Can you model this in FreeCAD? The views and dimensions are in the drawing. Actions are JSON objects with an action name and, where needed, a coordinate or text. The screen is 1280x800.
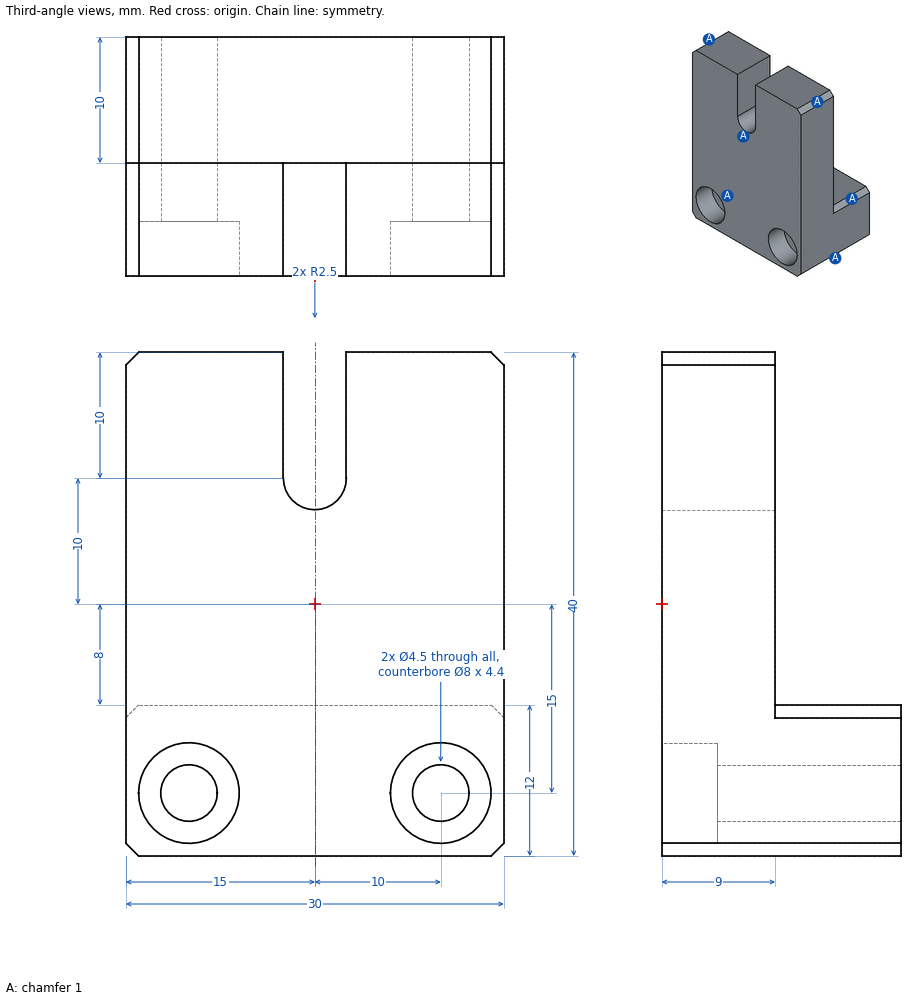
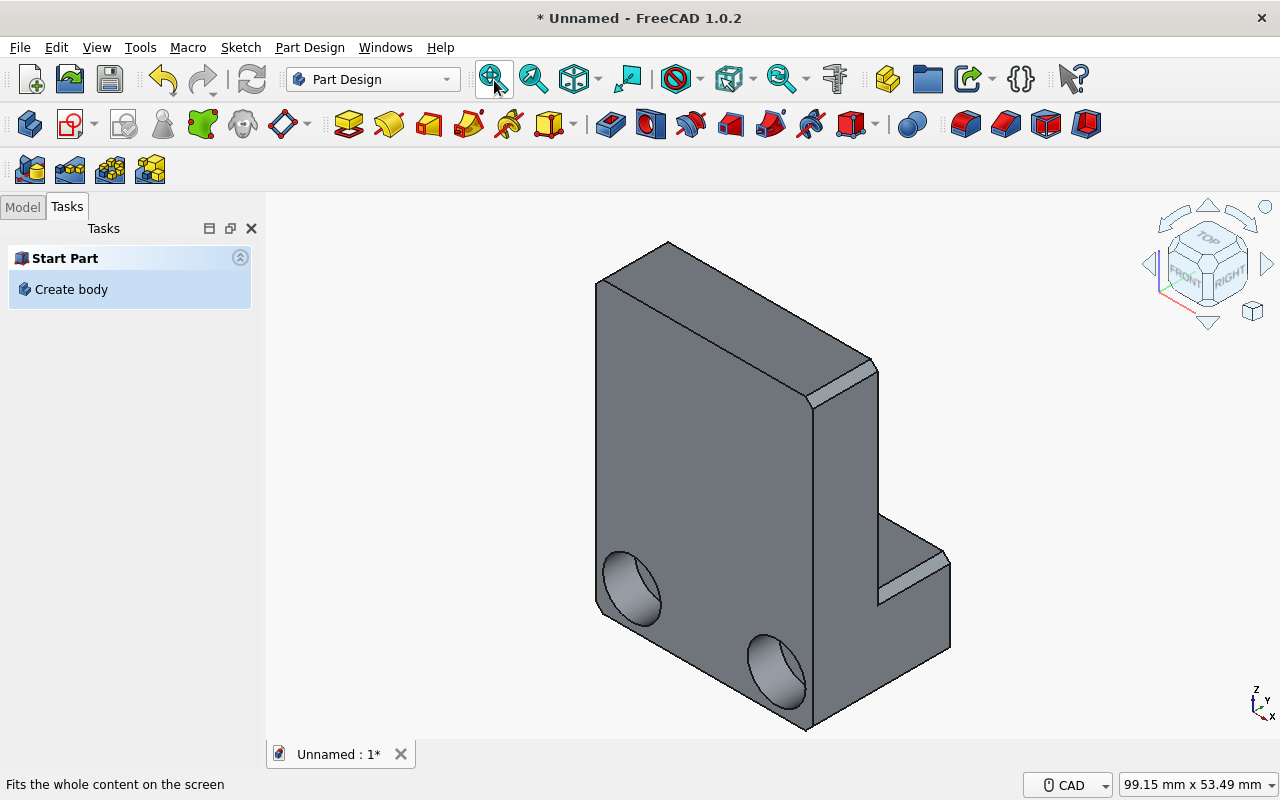
{"action": "left_click", "coordinate": [704, 456]}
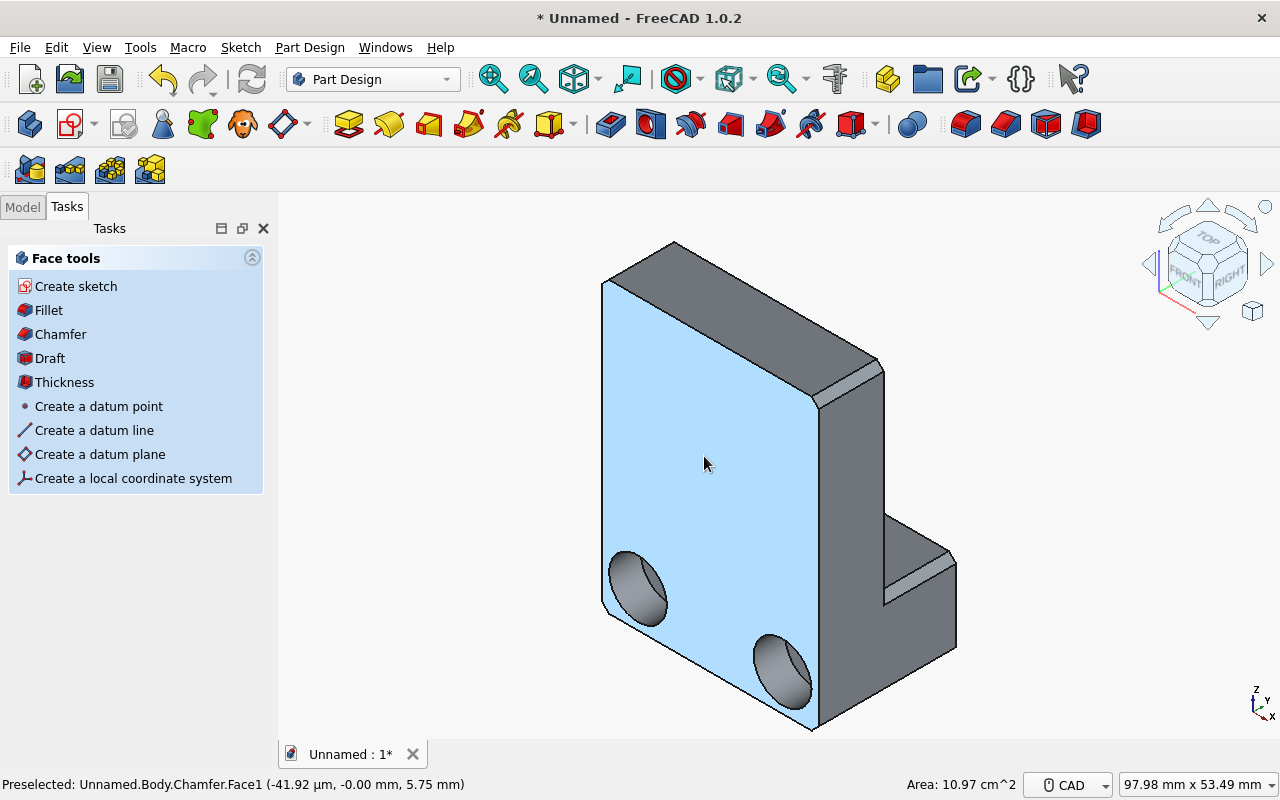
{"action": "left_click", "coordinate": [70, 124]}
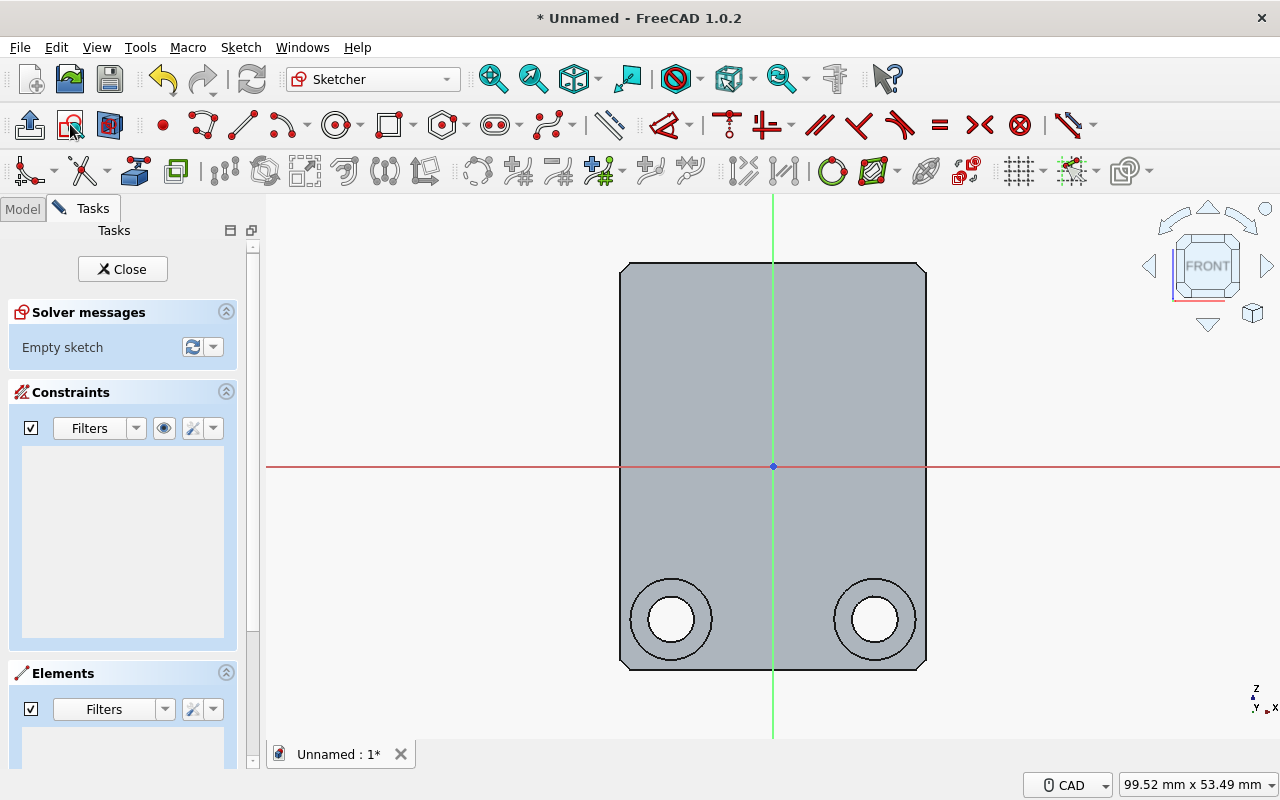
{"action": "scroll", "coordinate": [395, 711], "scroll_direction": "down", "scroll_amount": 1}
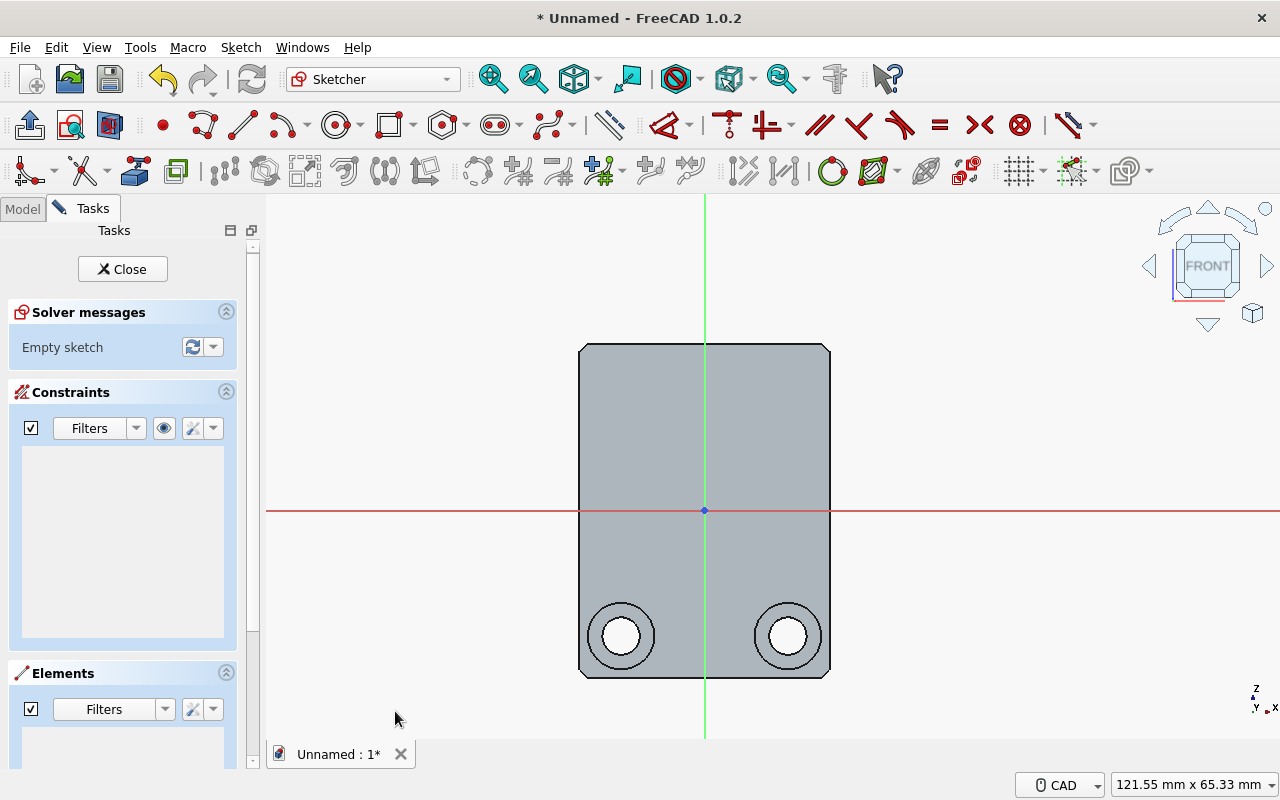
{"action": "scroll", "coordinate": [705, 357], "scroll_direction": "up", "scroll_amount": 3}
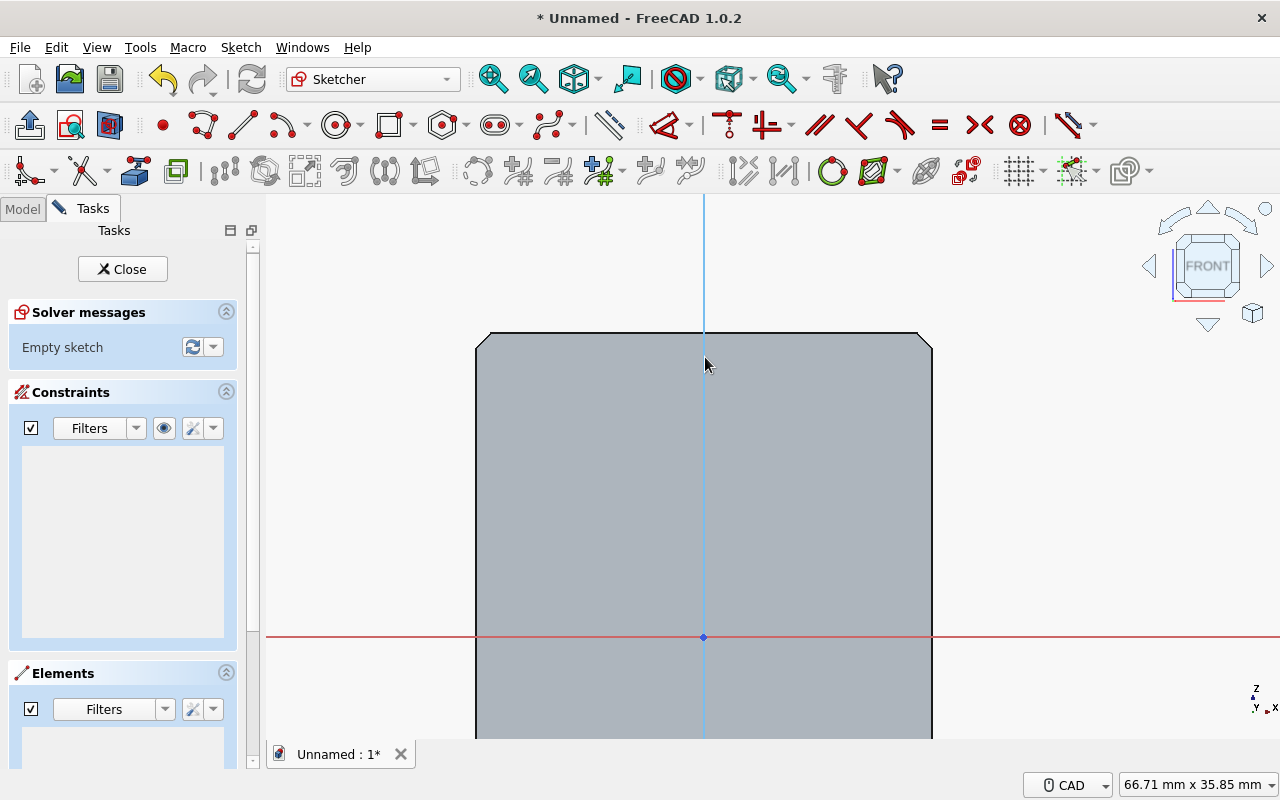
{"action": "left_click", "coordinate": [496, 126]}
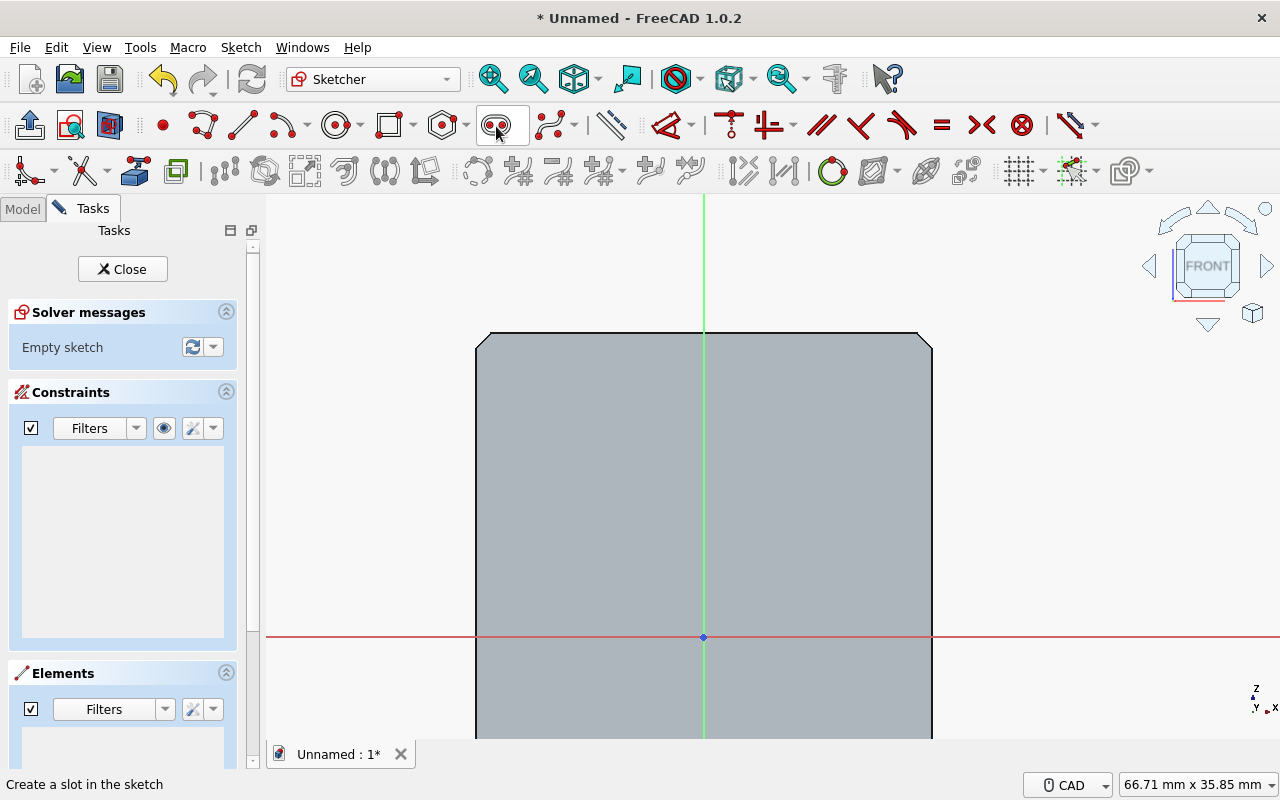
{"action": "left_click", "coordinate": [704, 485]}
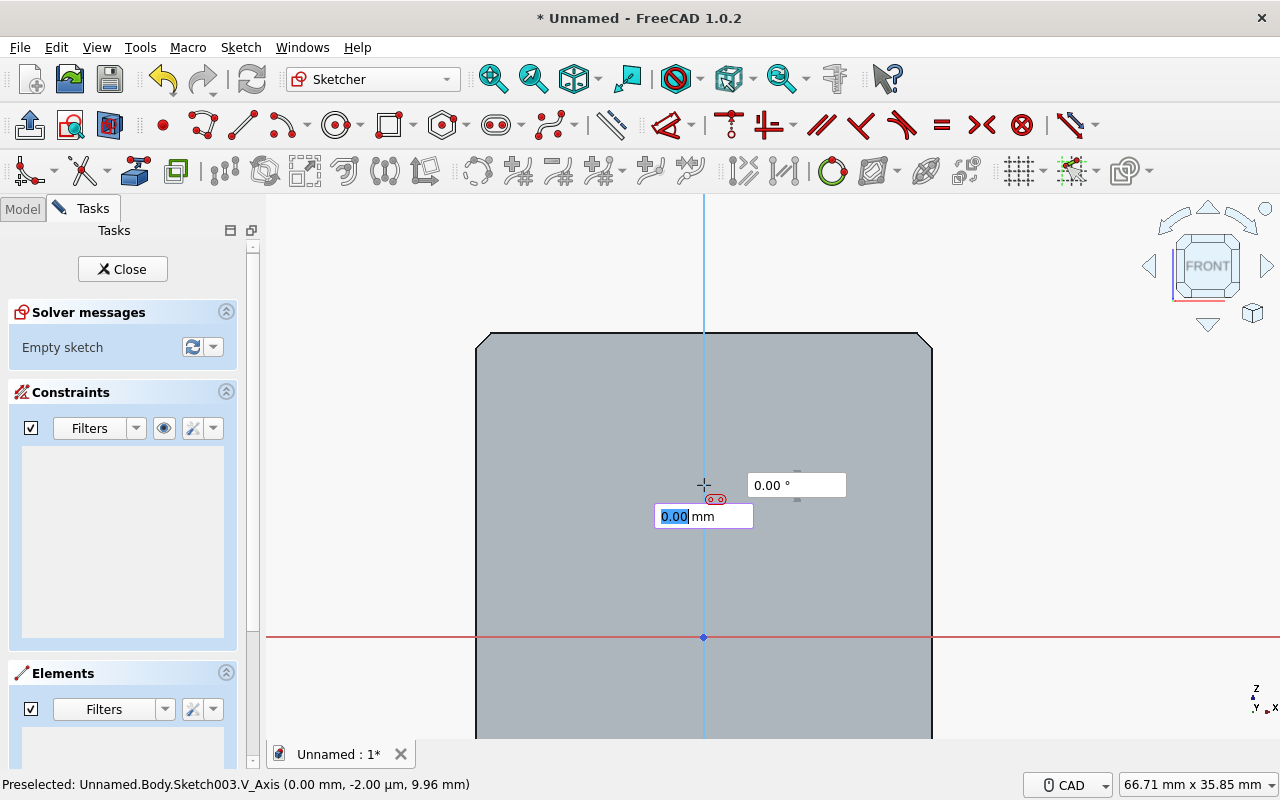
{"action": "left_click", "coordinate": [713, 333]}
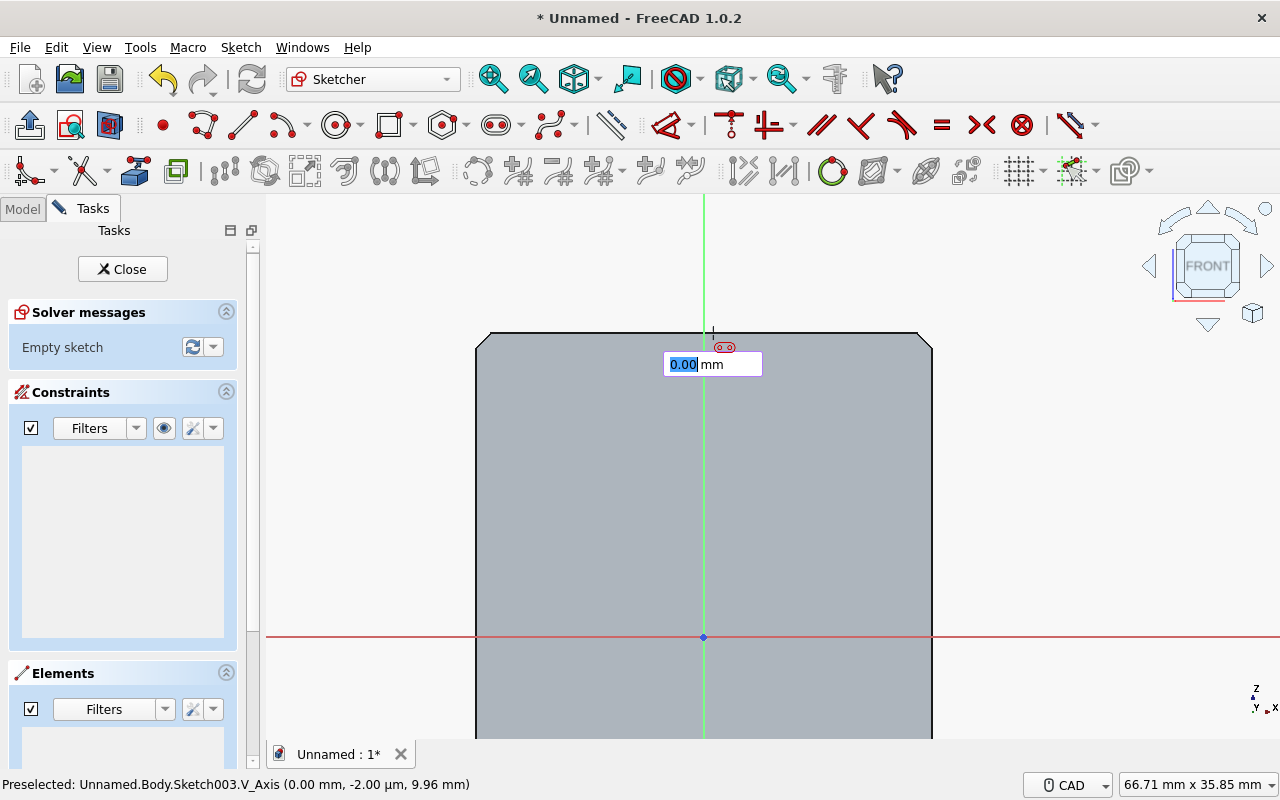
{"action": "left_click", "coordinate": [742, 409]}
{"action": "key", "text": "Escape"}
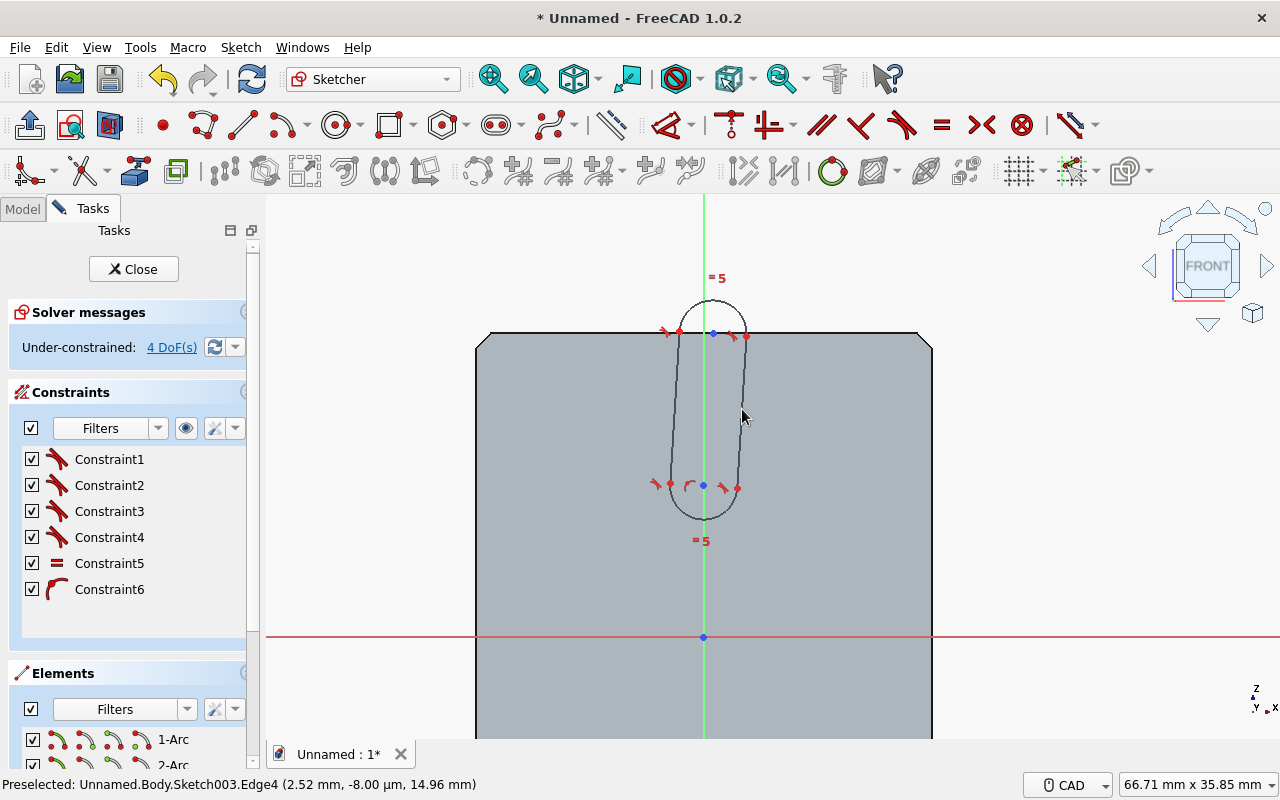
{"action": "left_click", "coordinate": [673, 438]}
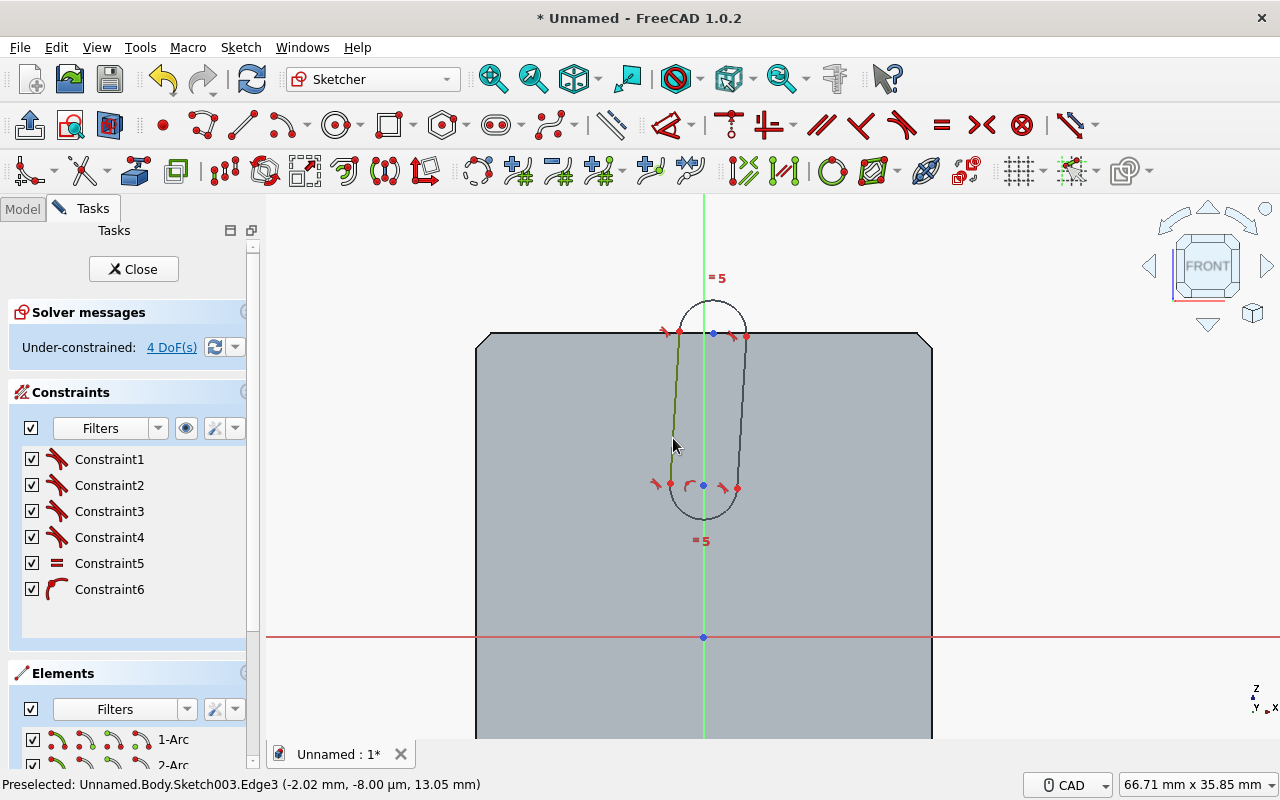
{"action": "left_click", "coordinate": [796, 126]}